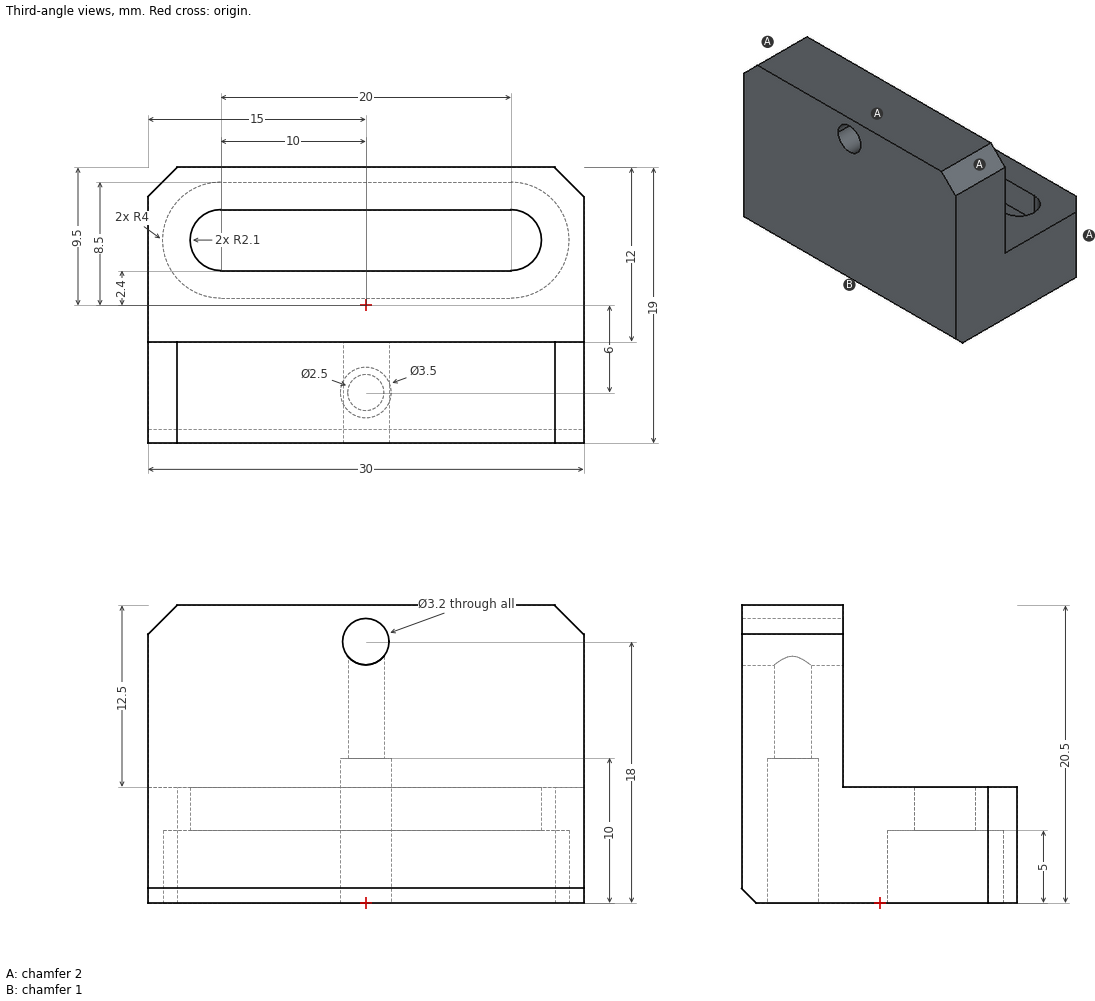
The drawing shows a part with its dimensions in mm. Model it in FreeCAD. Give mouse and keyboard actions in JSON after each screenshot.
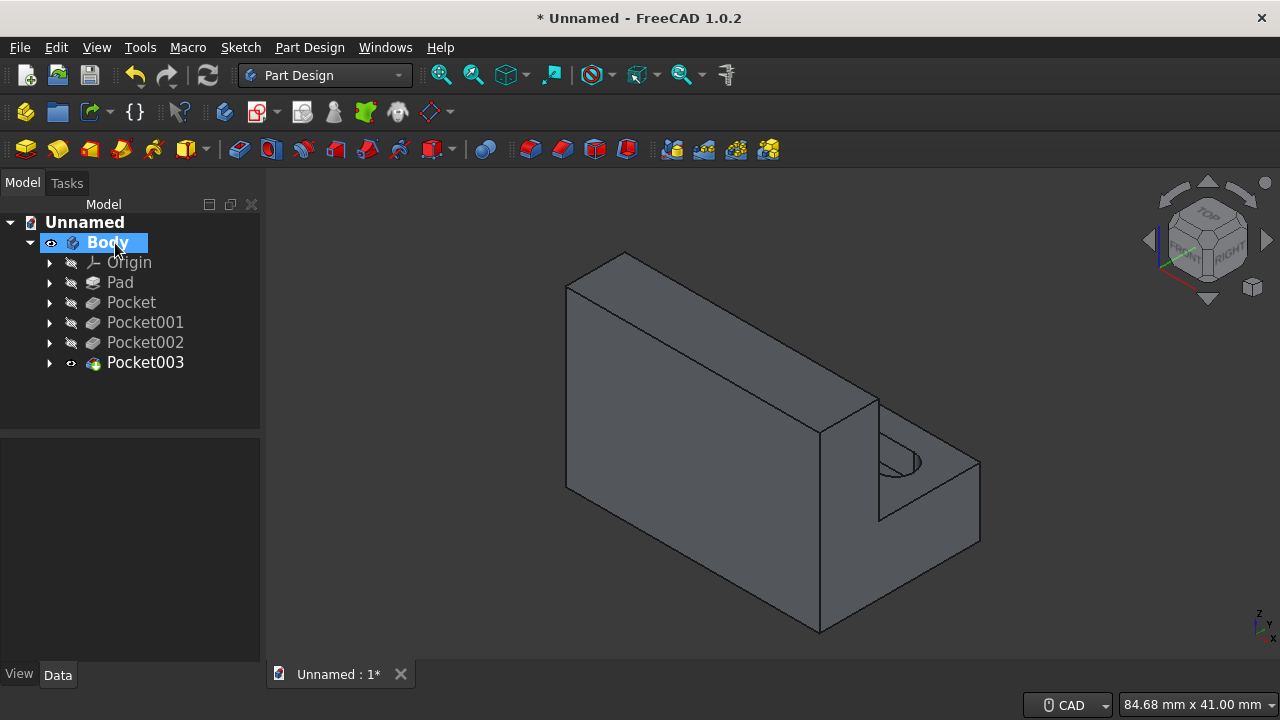
{"action": "left_click", "coordinate": [729, 480]}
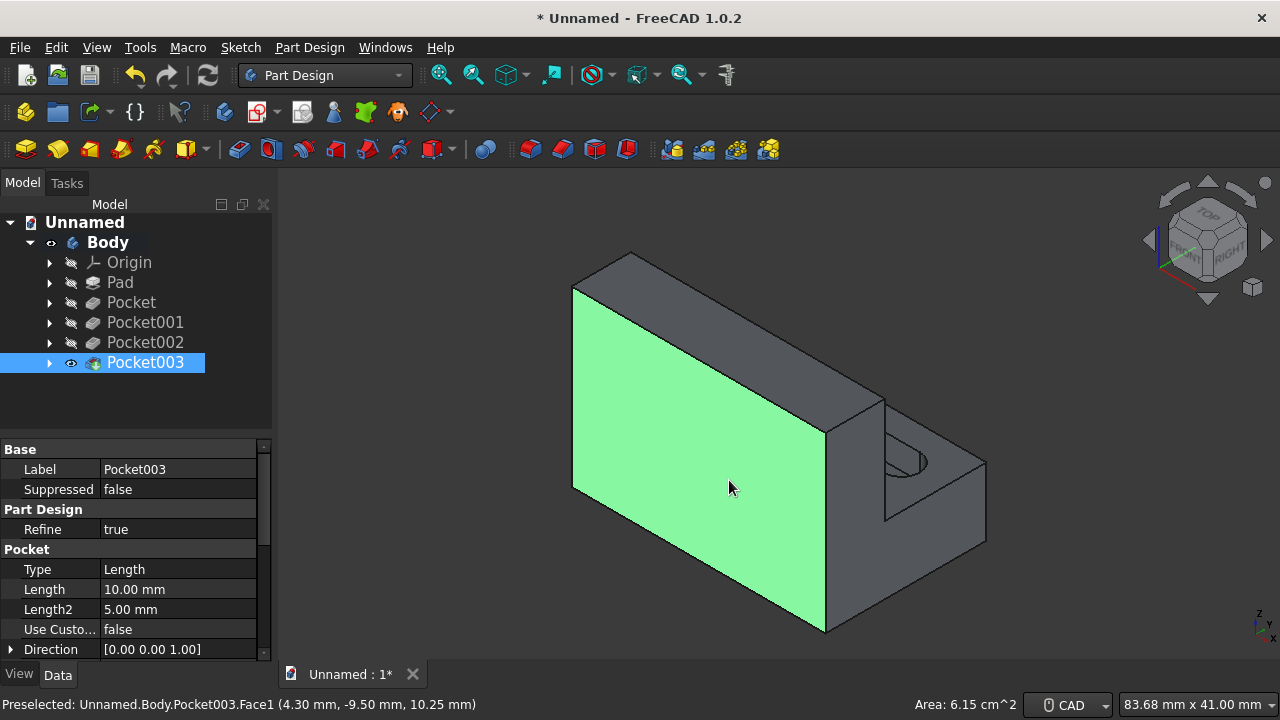
{"action": "left_click", "coordinate": [258, 112]}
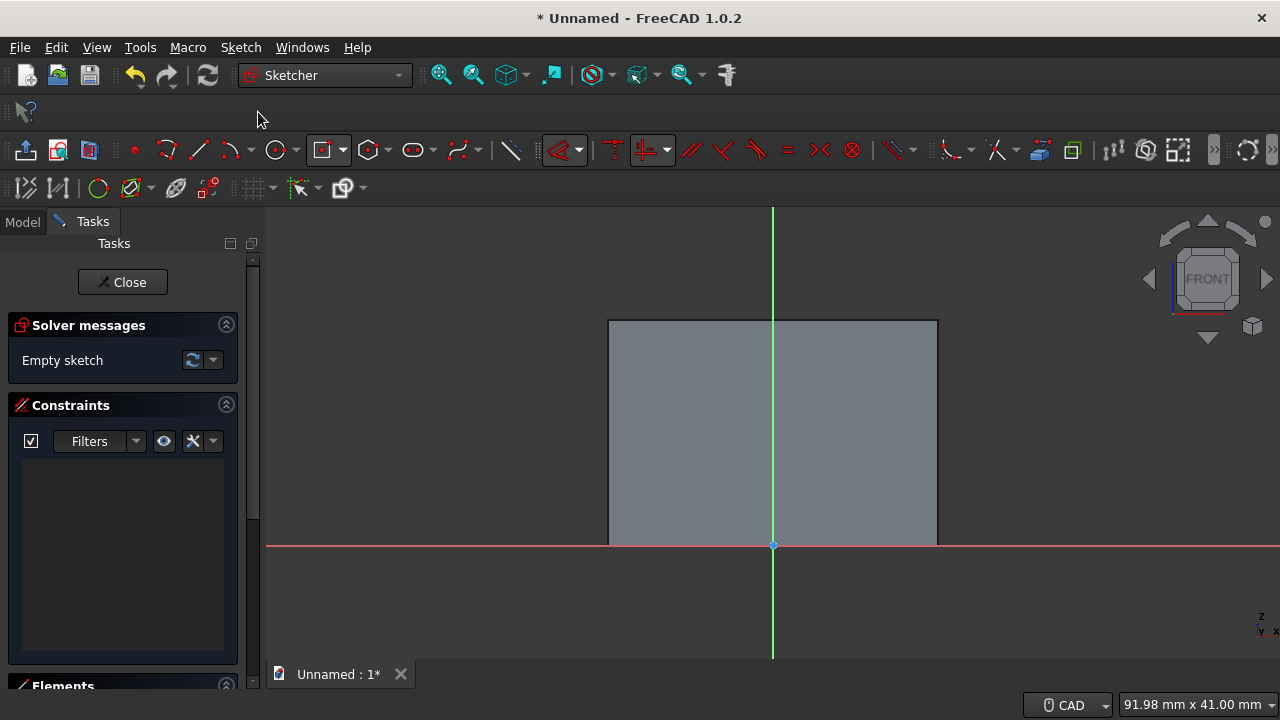
{"action": "scroll", "coordinate": [784, 334], "scroll_direction": "up", "scroll_amount": 10}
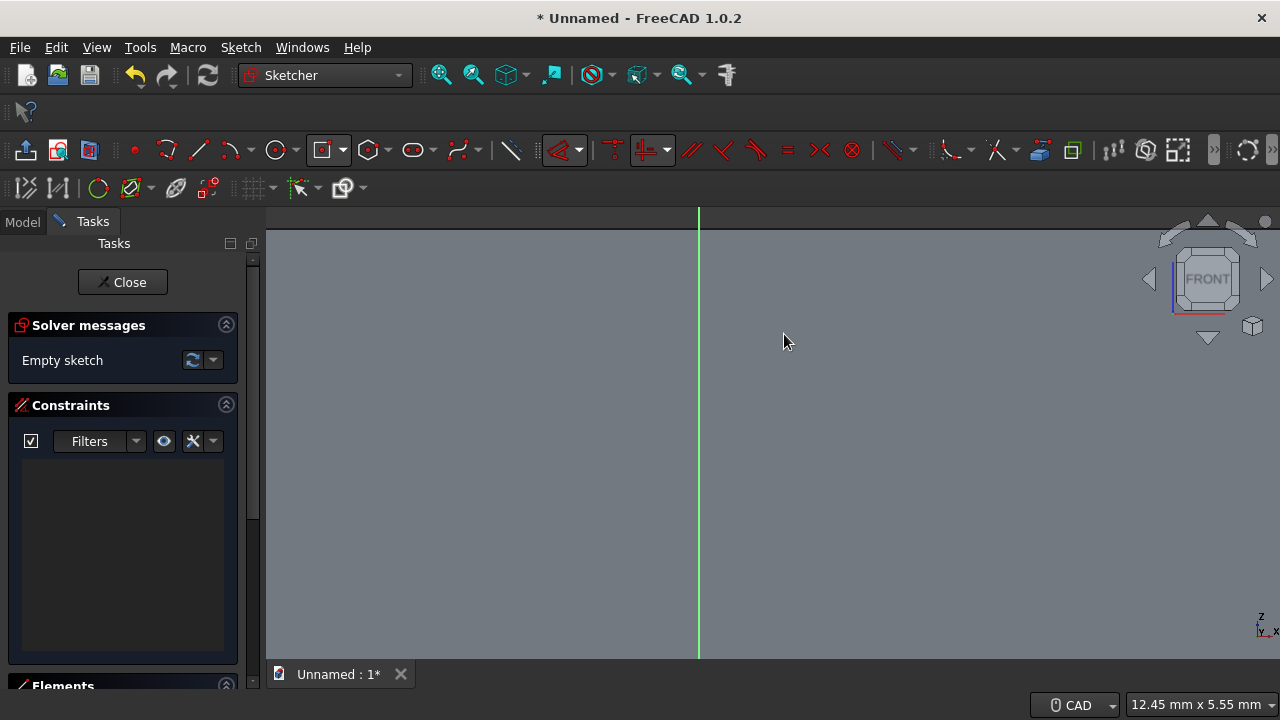
{"action": "left_click", "coordinate": [276, 150]}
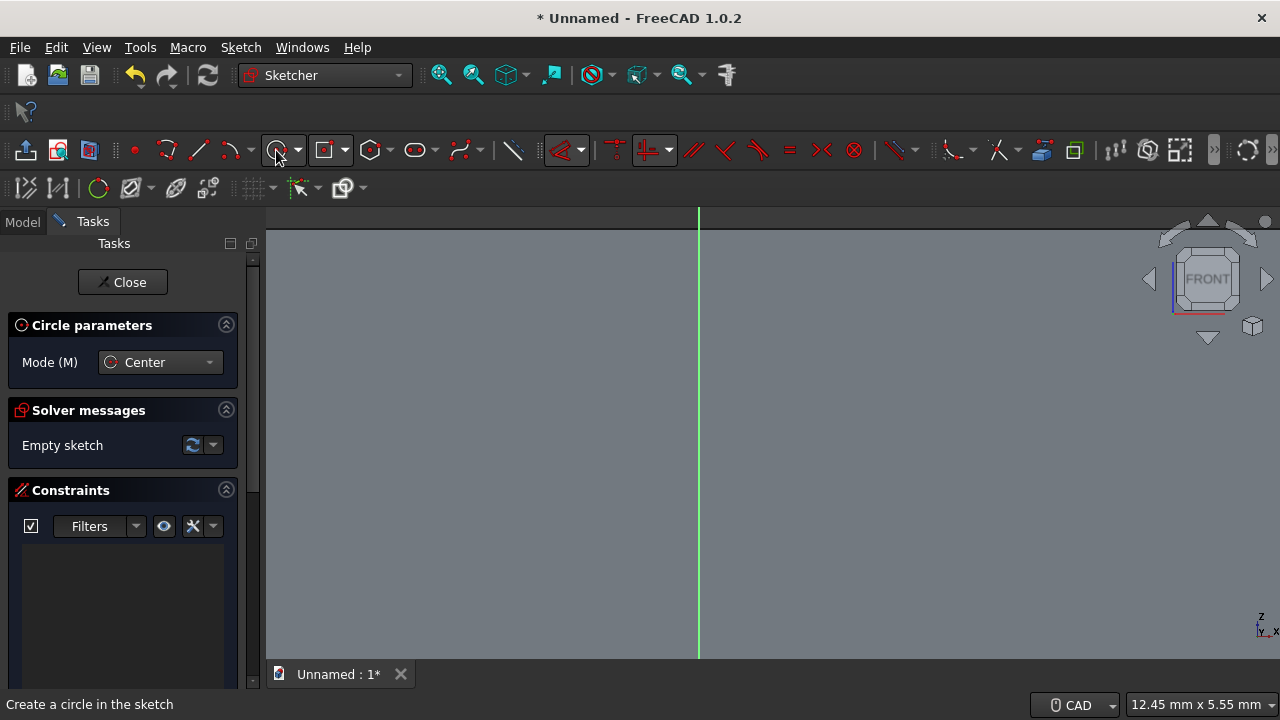
{"action": "left_click", "coordinate": [699, 432]}
{"action": "mouse_move", "coordinate": [792, 340]}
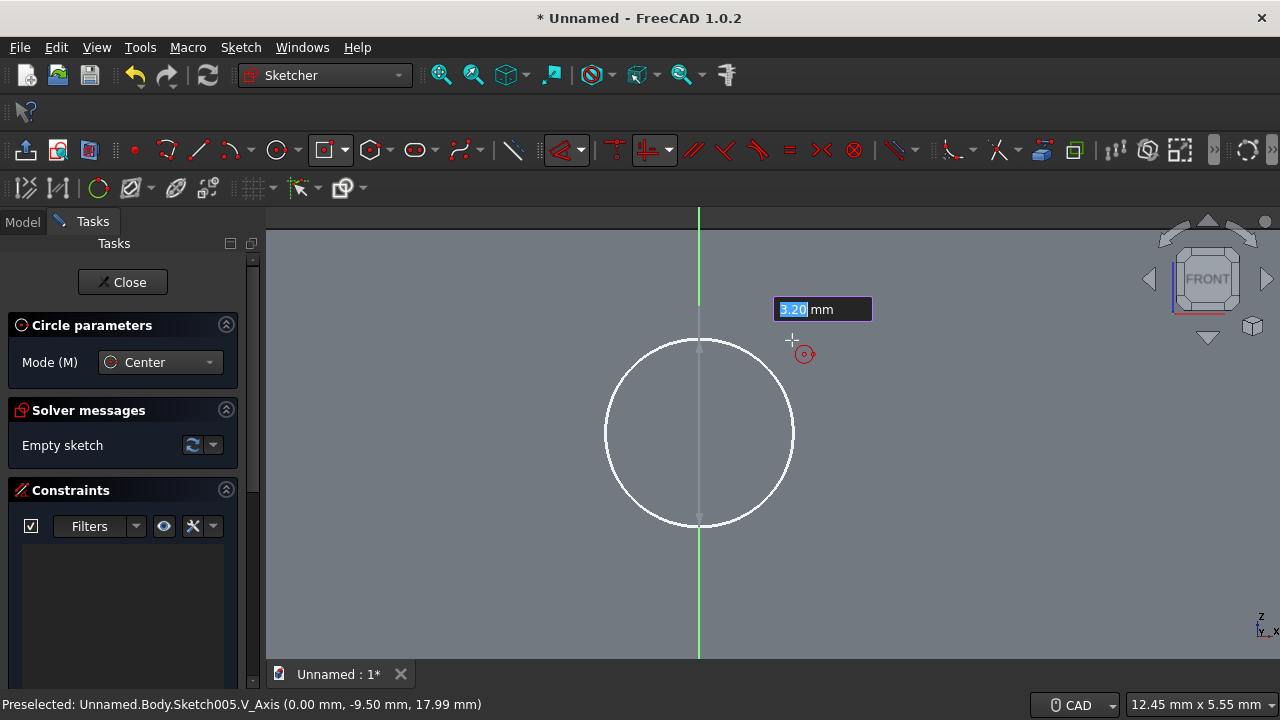
{"action": "type", "text": "3.2"}
{"action": "key", "text": "Return"}
{"action": "key", "text": "Escape"}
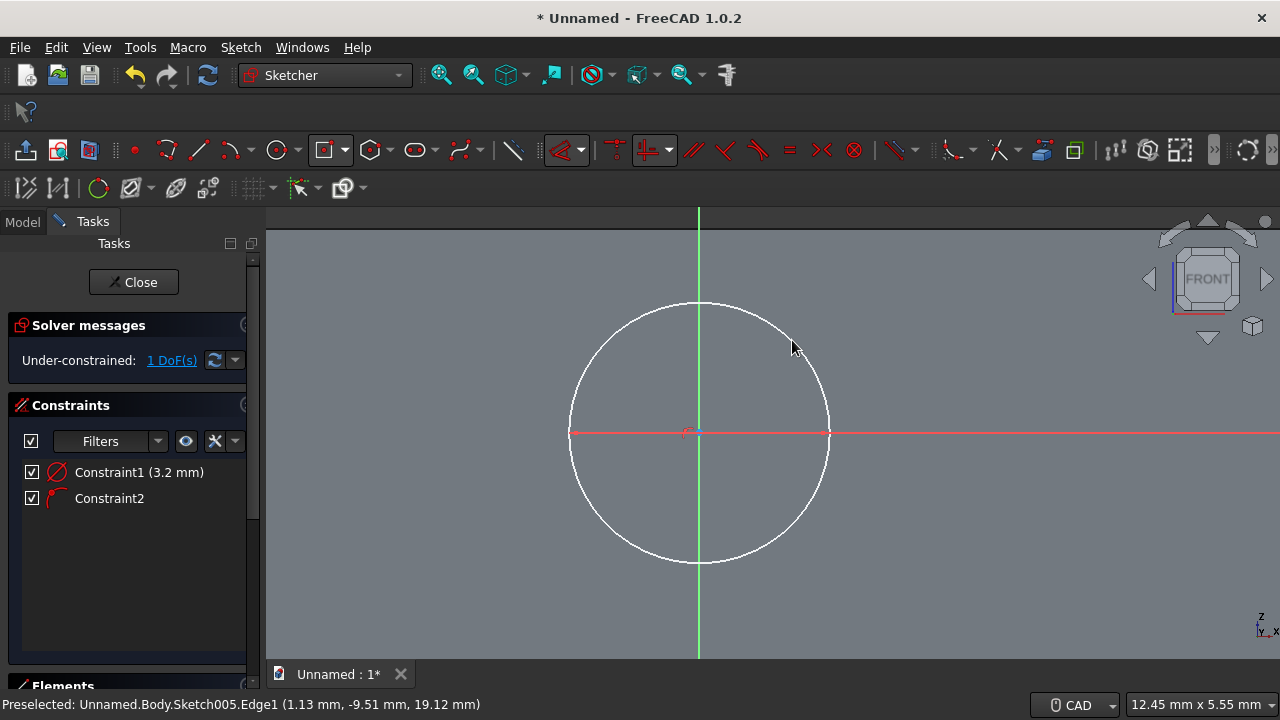
{"action": "left_click", "coordinate": [699, 433]}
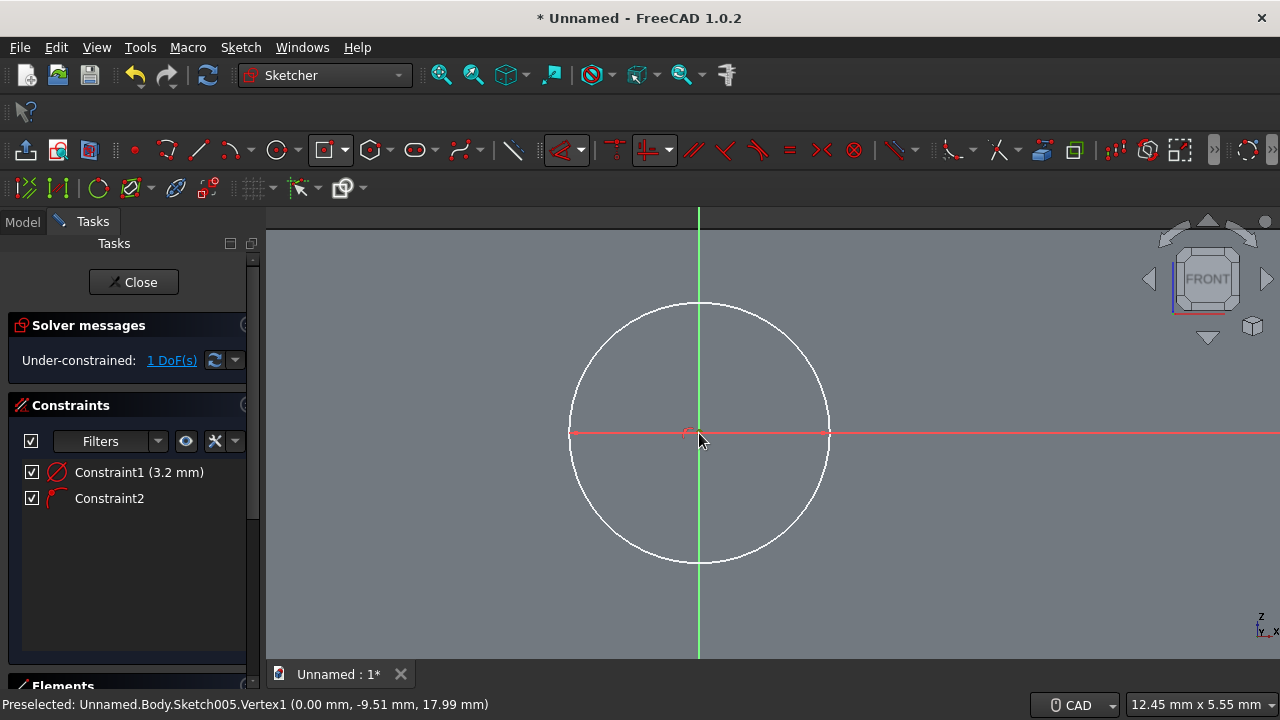
{"action": "key", "text": "i"}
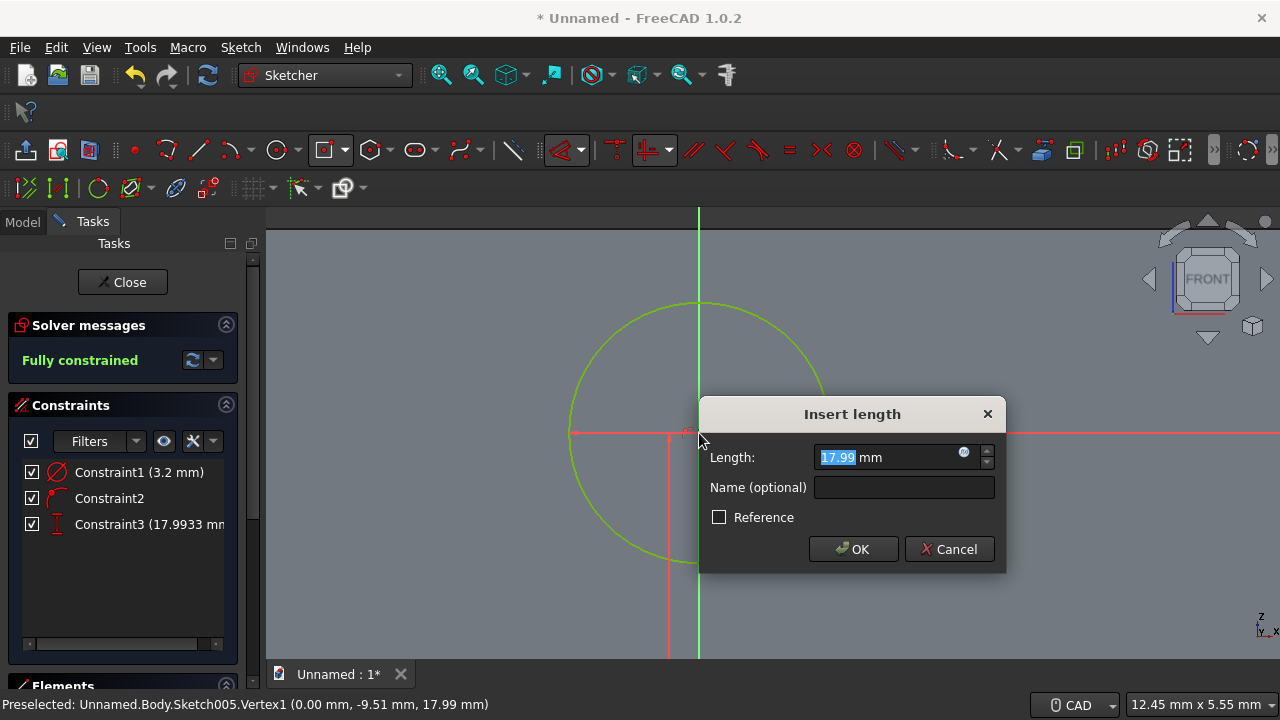
{"action": "type", "text": "18"}
{"action": "key", "text": "Return"}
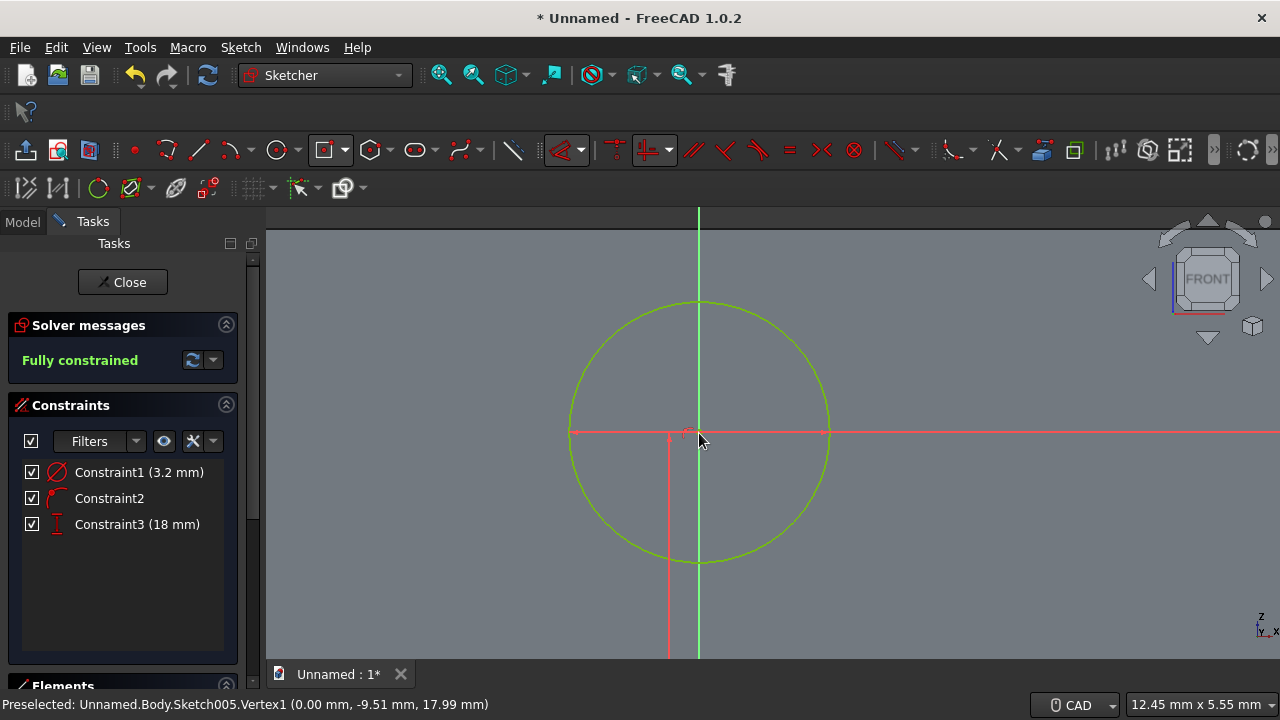
{"action": "left_click", "coordinate": [123, 282]}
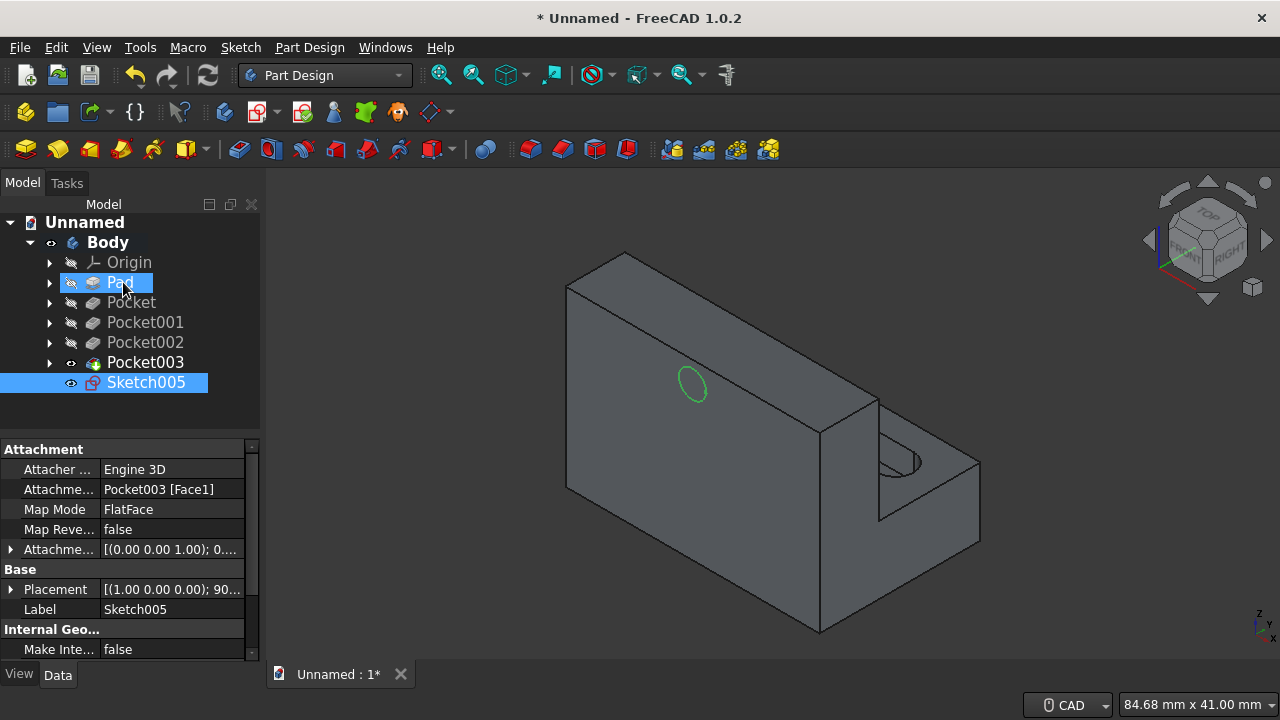
{"action": "left_click", "coordinate": [272, 150]}